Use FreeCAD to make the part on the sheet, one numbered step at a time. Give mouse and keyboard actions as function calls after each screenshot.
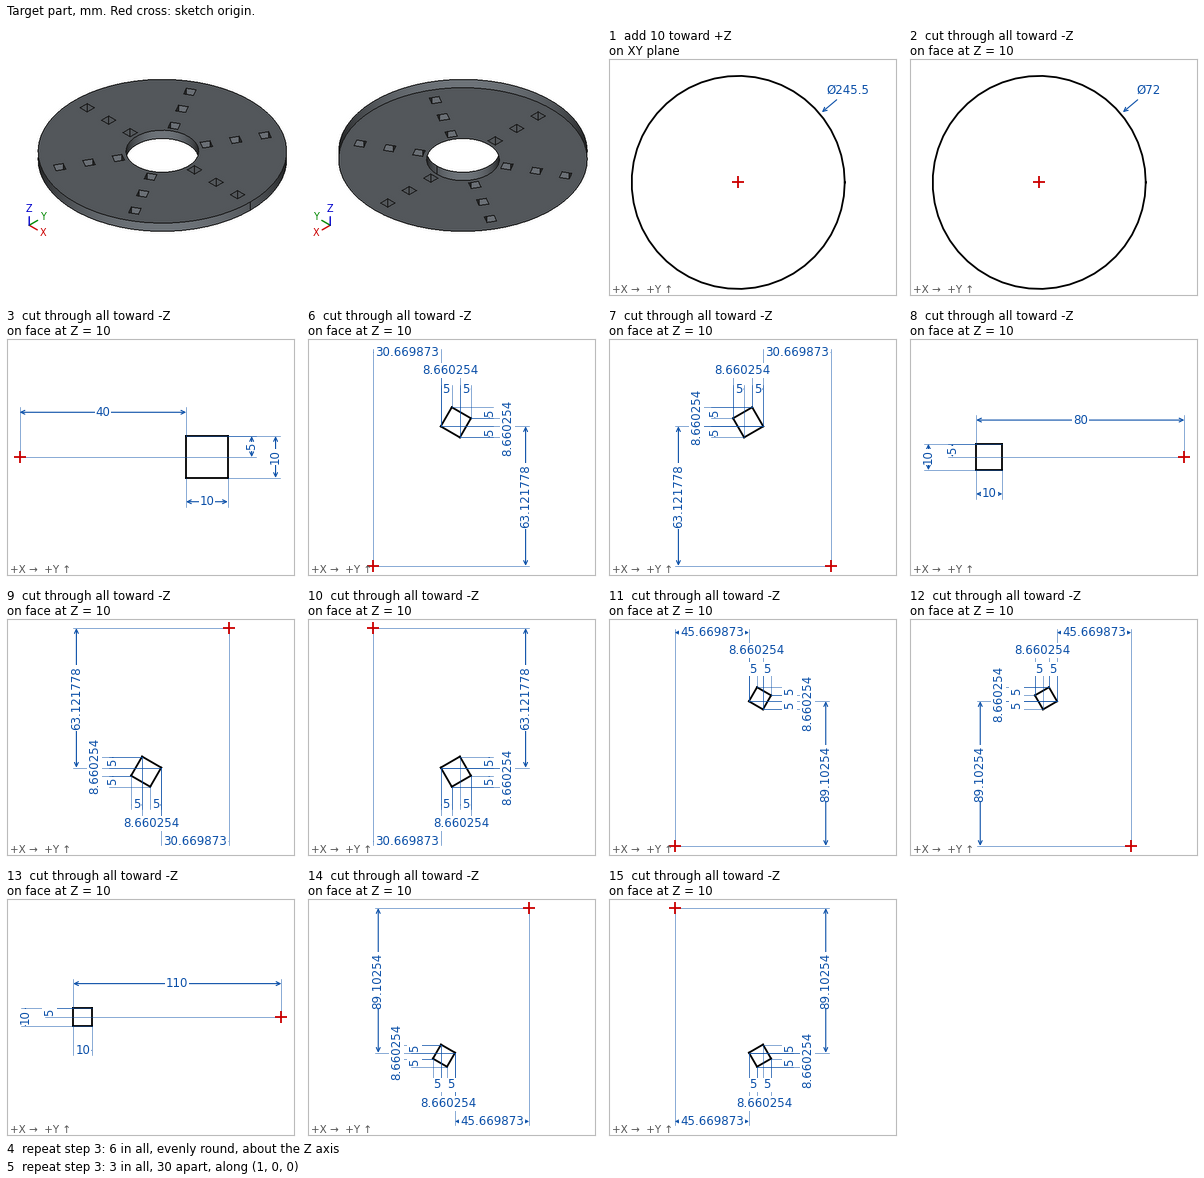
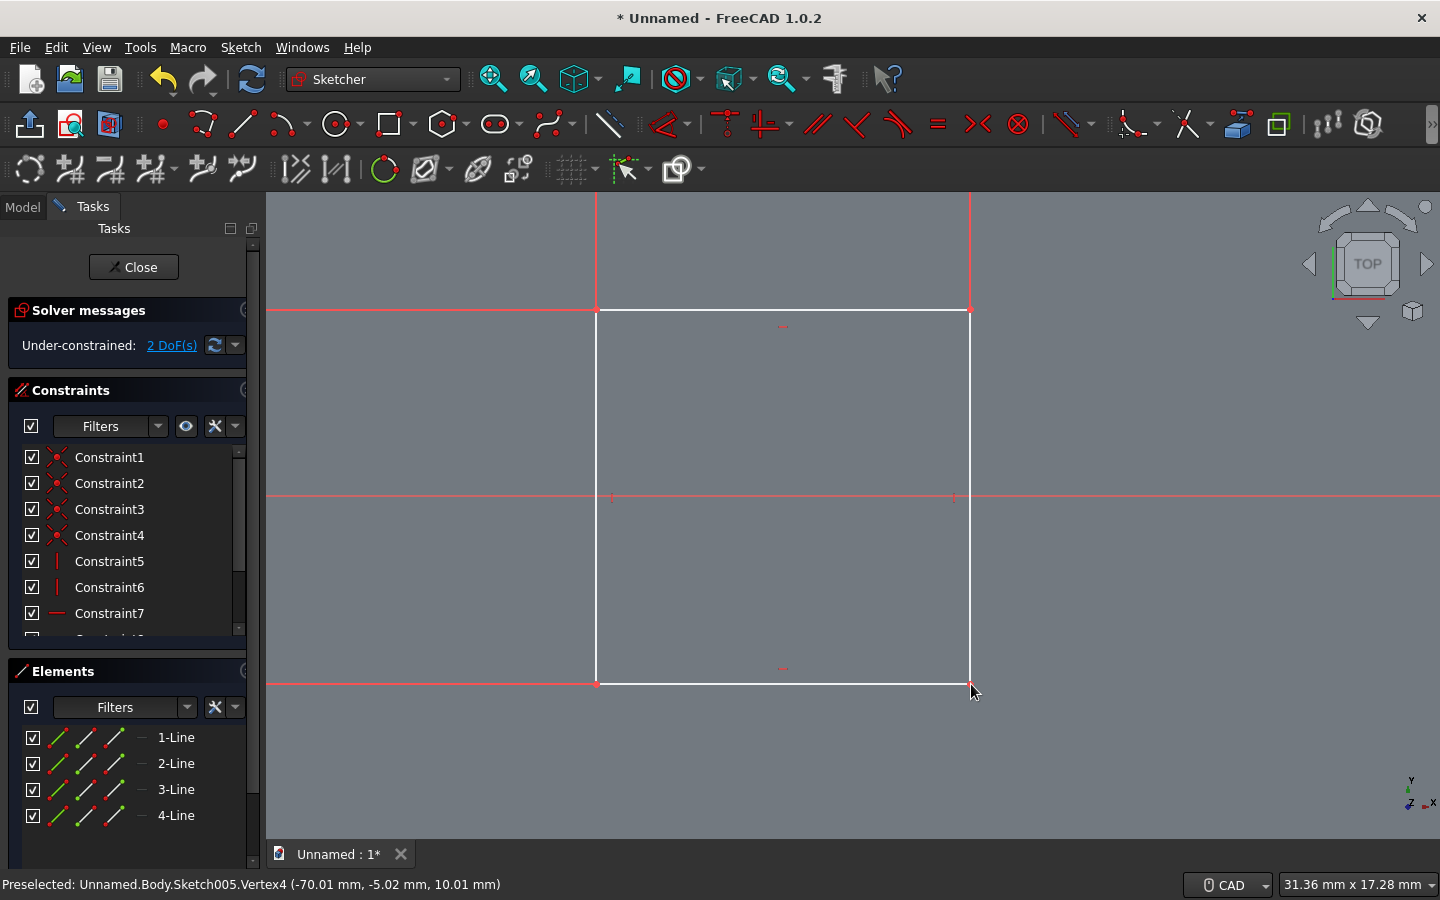
key(d)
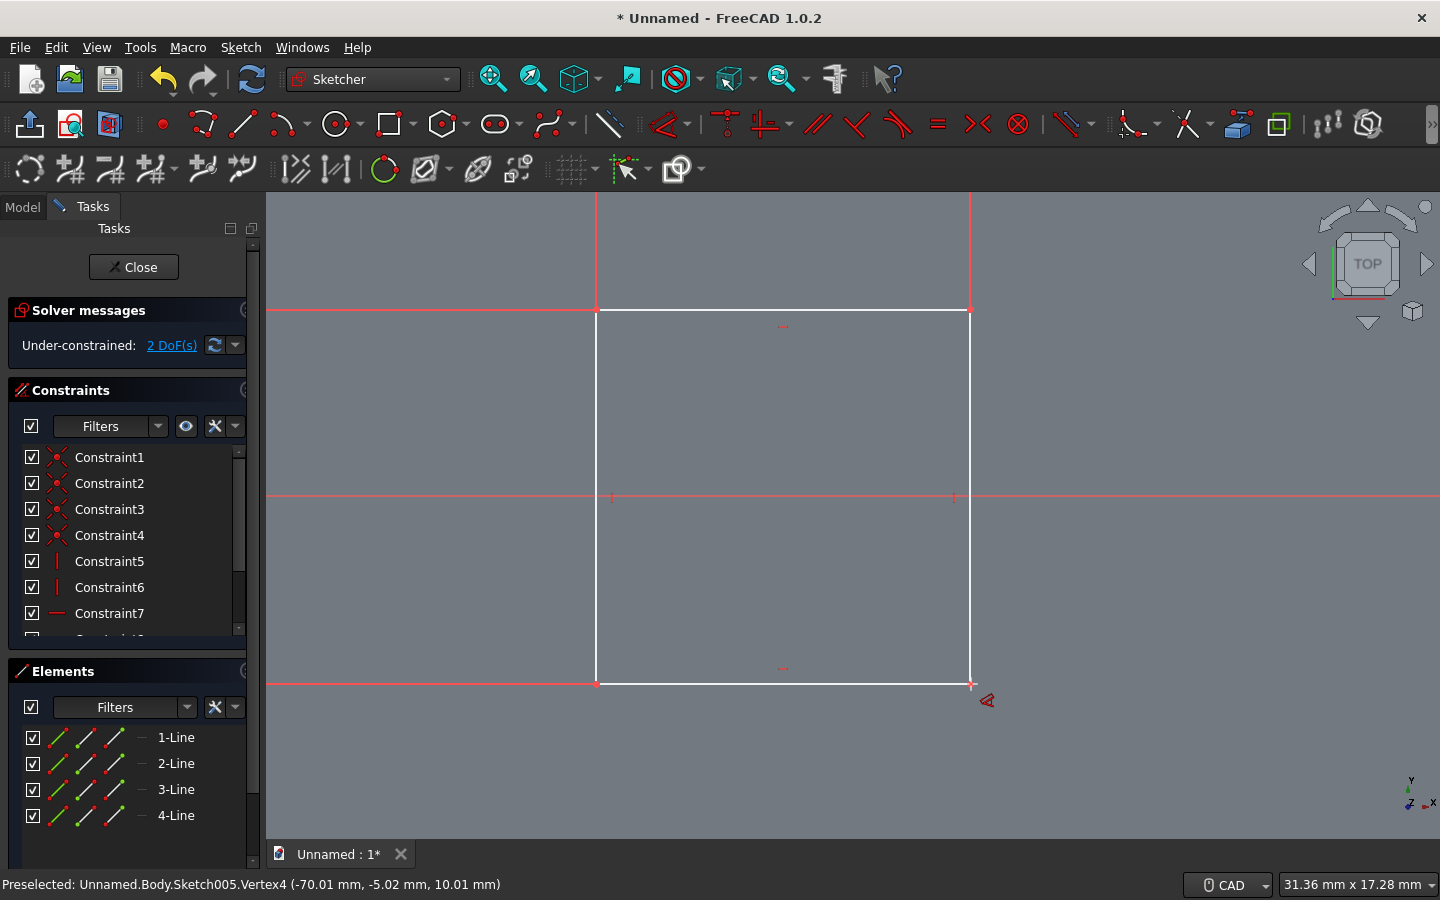
click(596, 310)
click(562, 403)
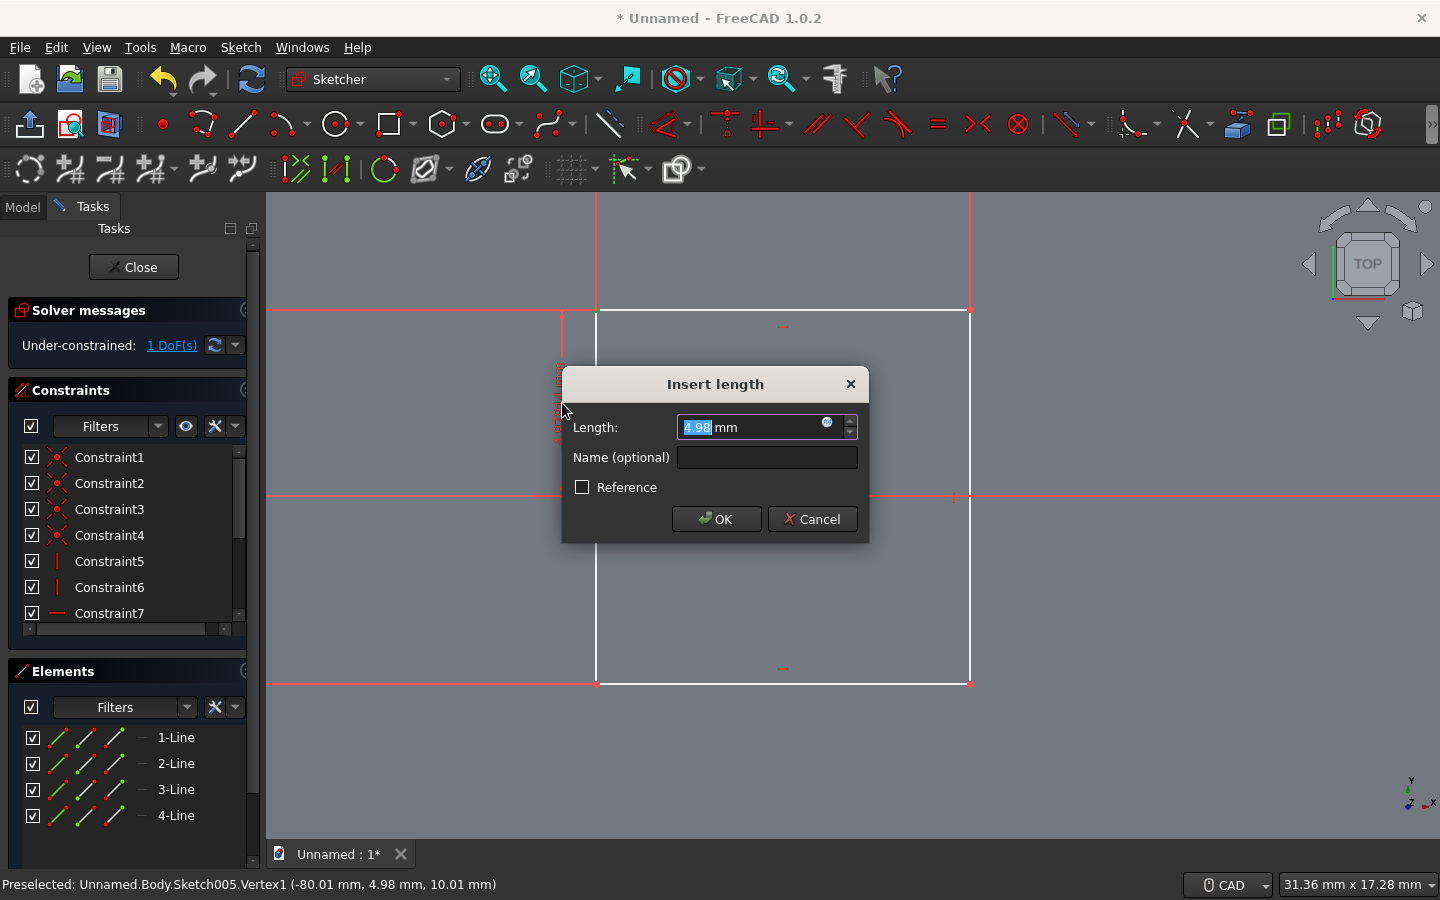
text(5)
key(Return)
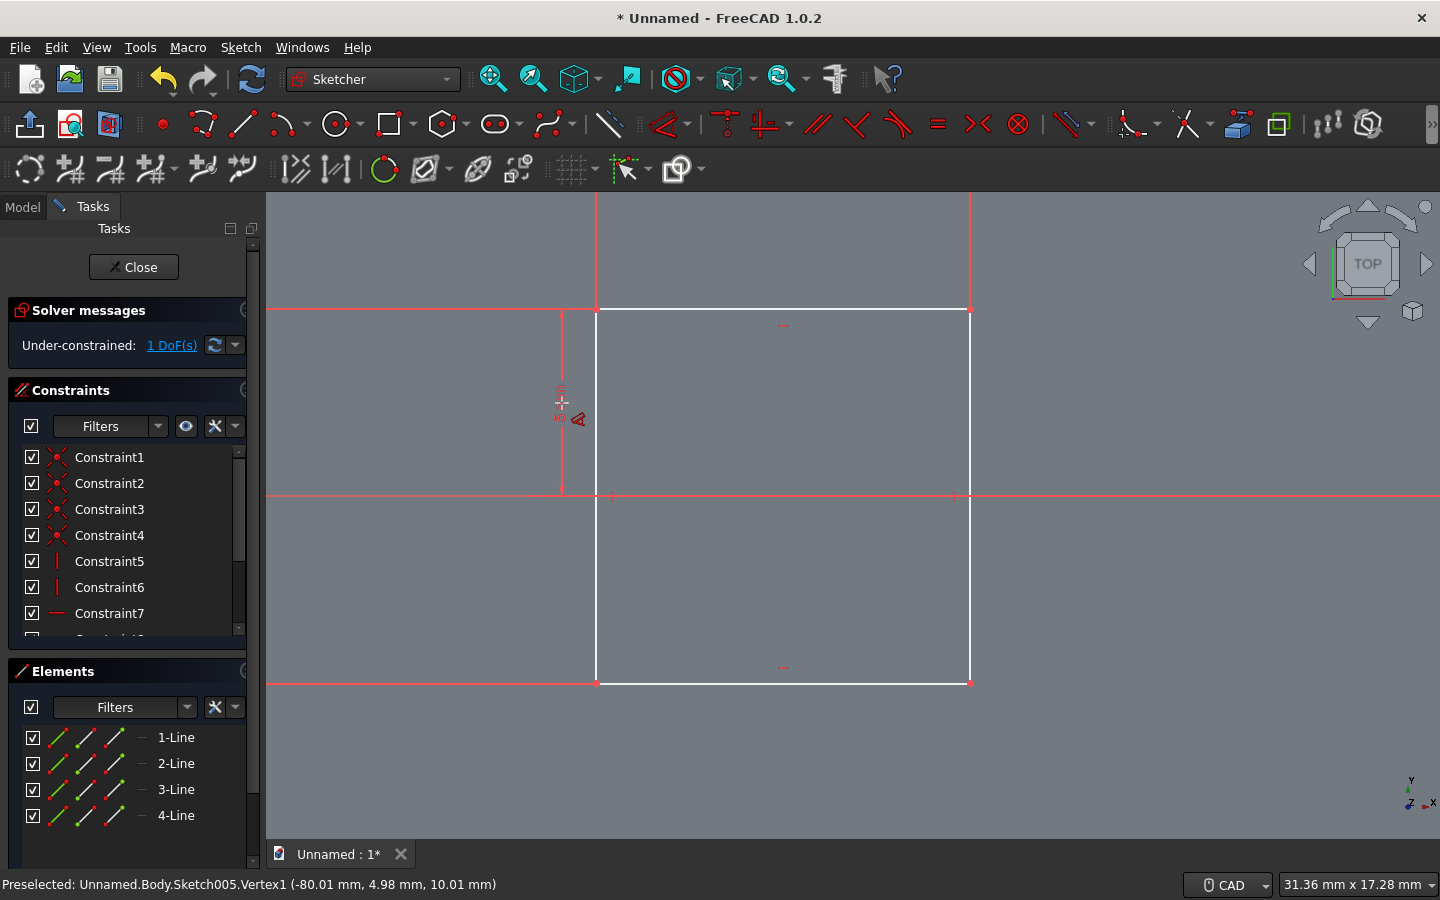
click(596, 309)
click(936, 275)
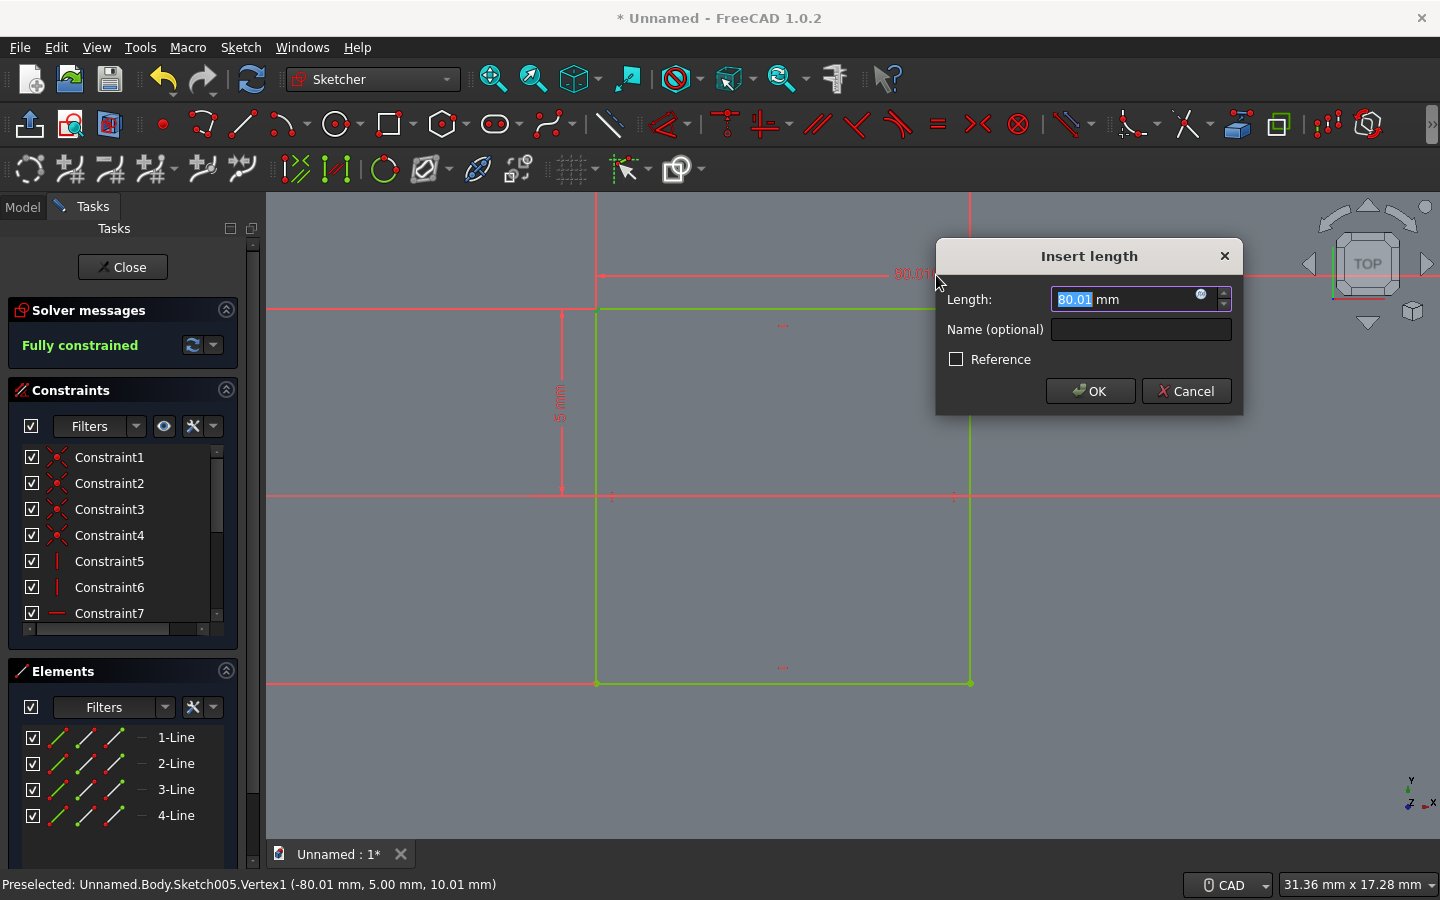
text(80)
key(Return)
key(Escape)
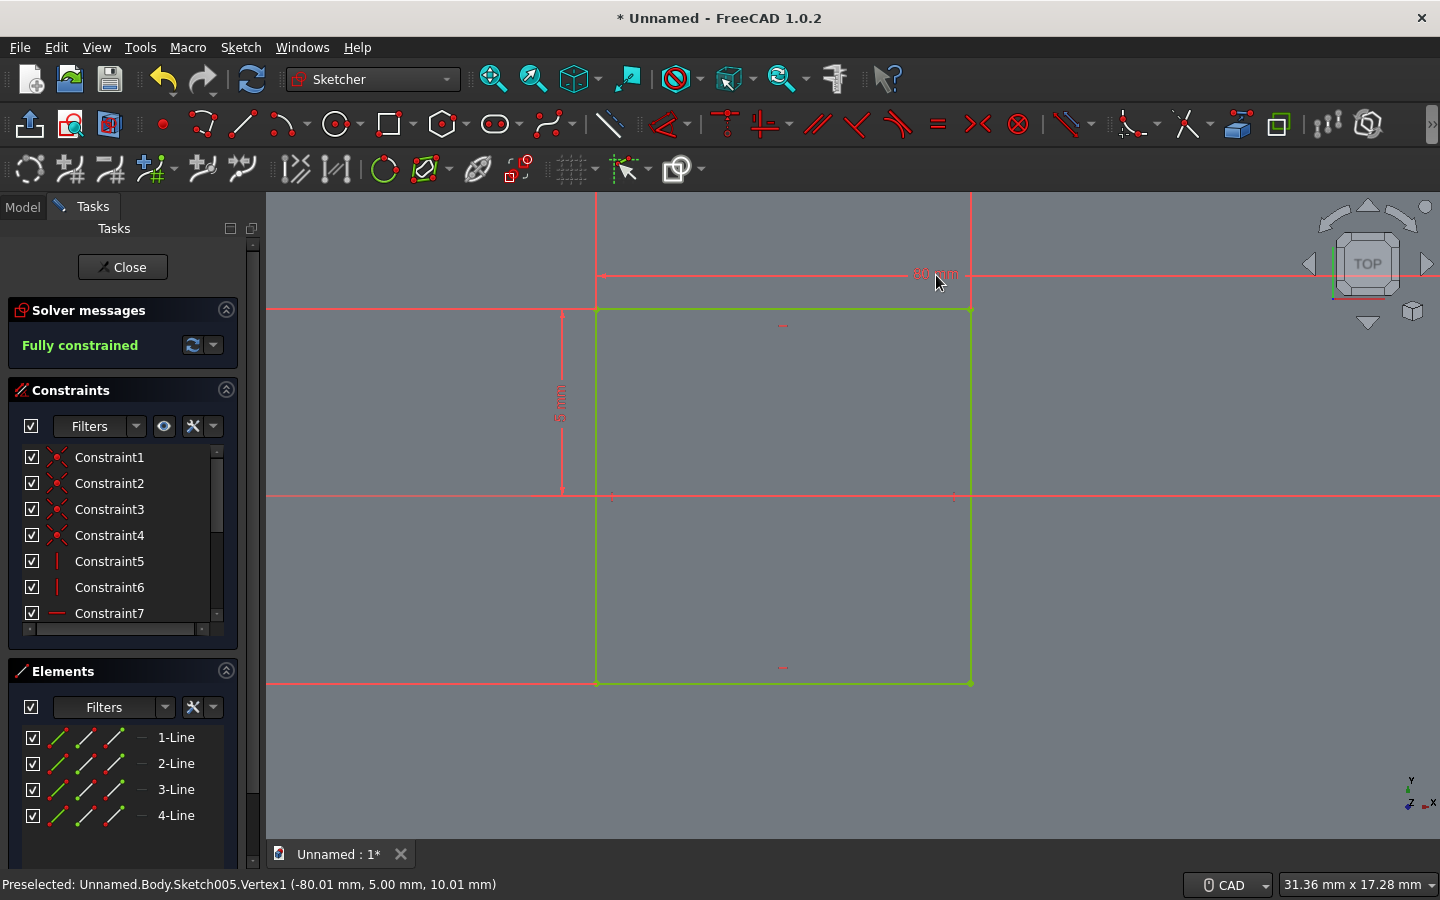
click(123, 267)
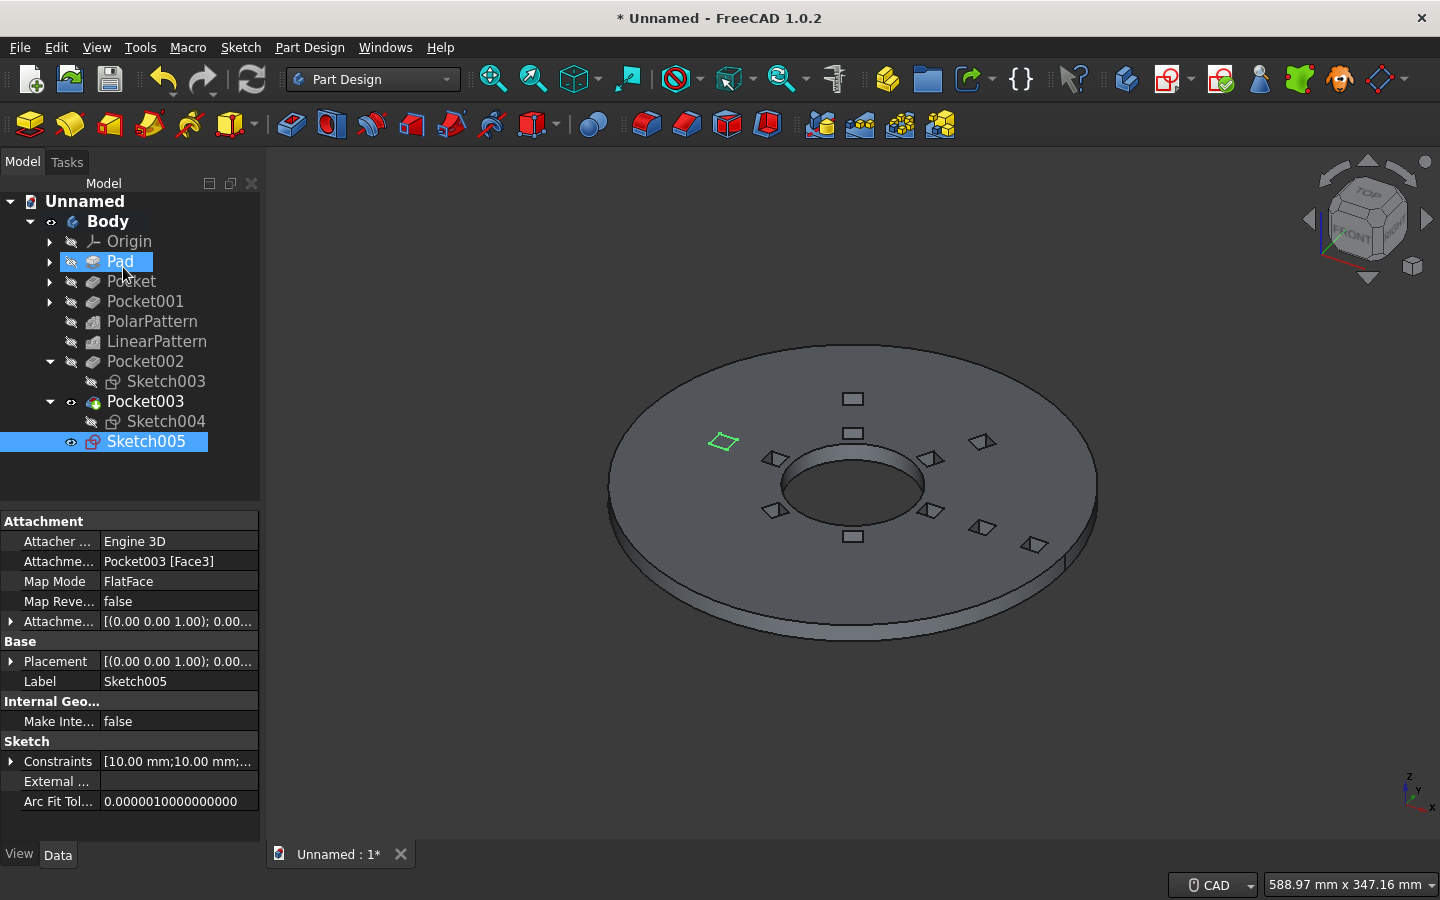
click(292, 124)